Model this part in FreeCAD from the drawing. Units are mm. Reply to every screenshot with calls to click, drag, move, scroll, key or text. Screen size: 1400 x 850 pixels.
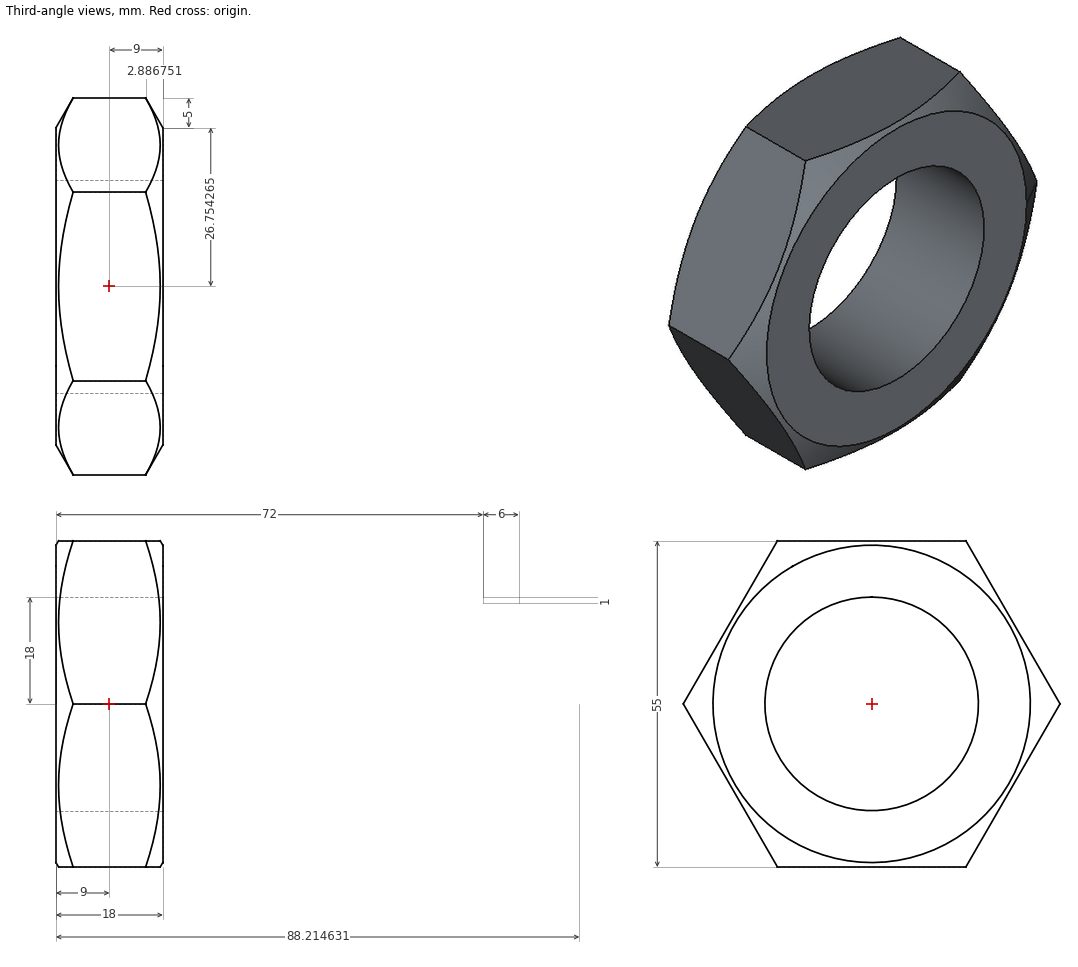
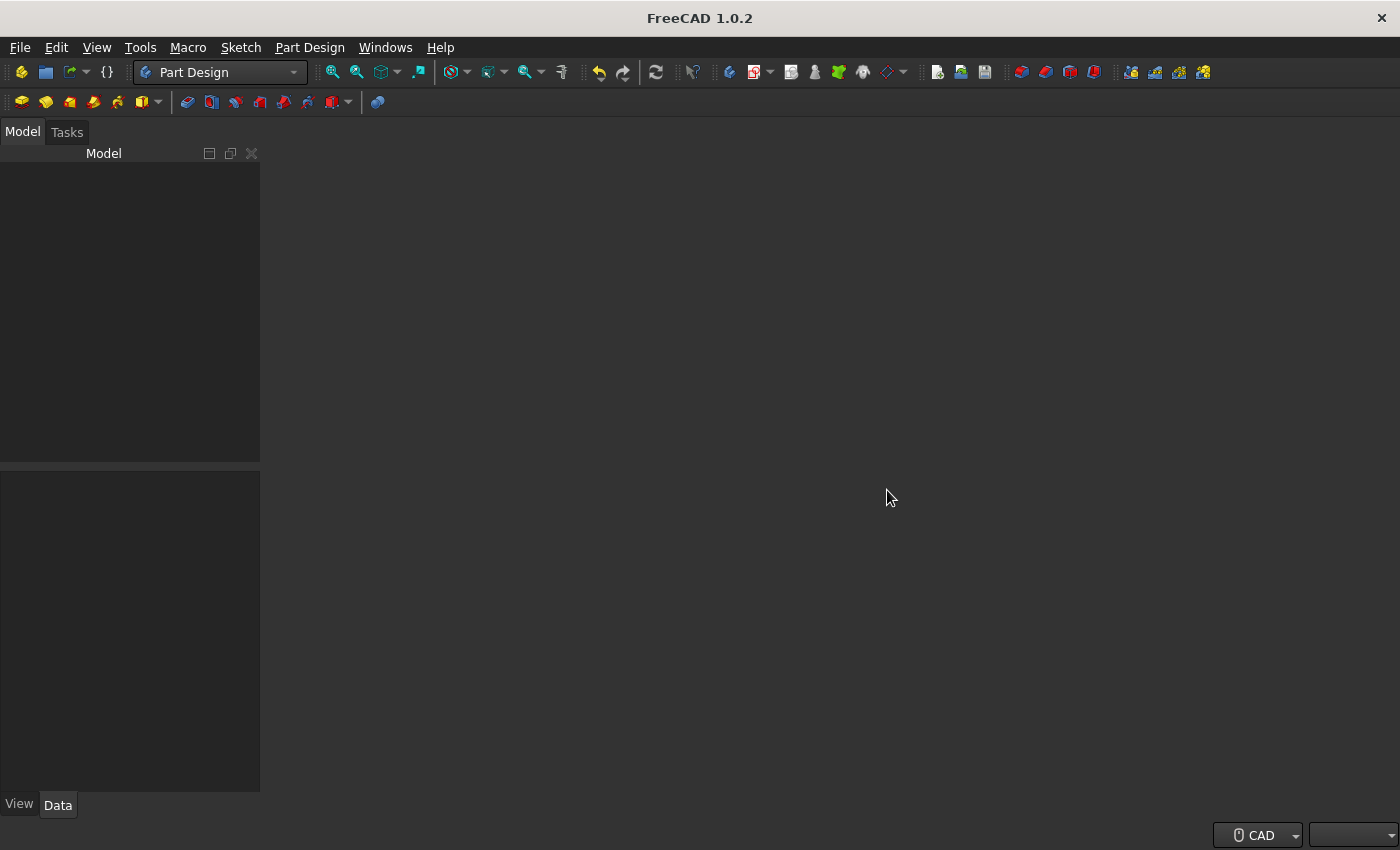
key(ctrl+n)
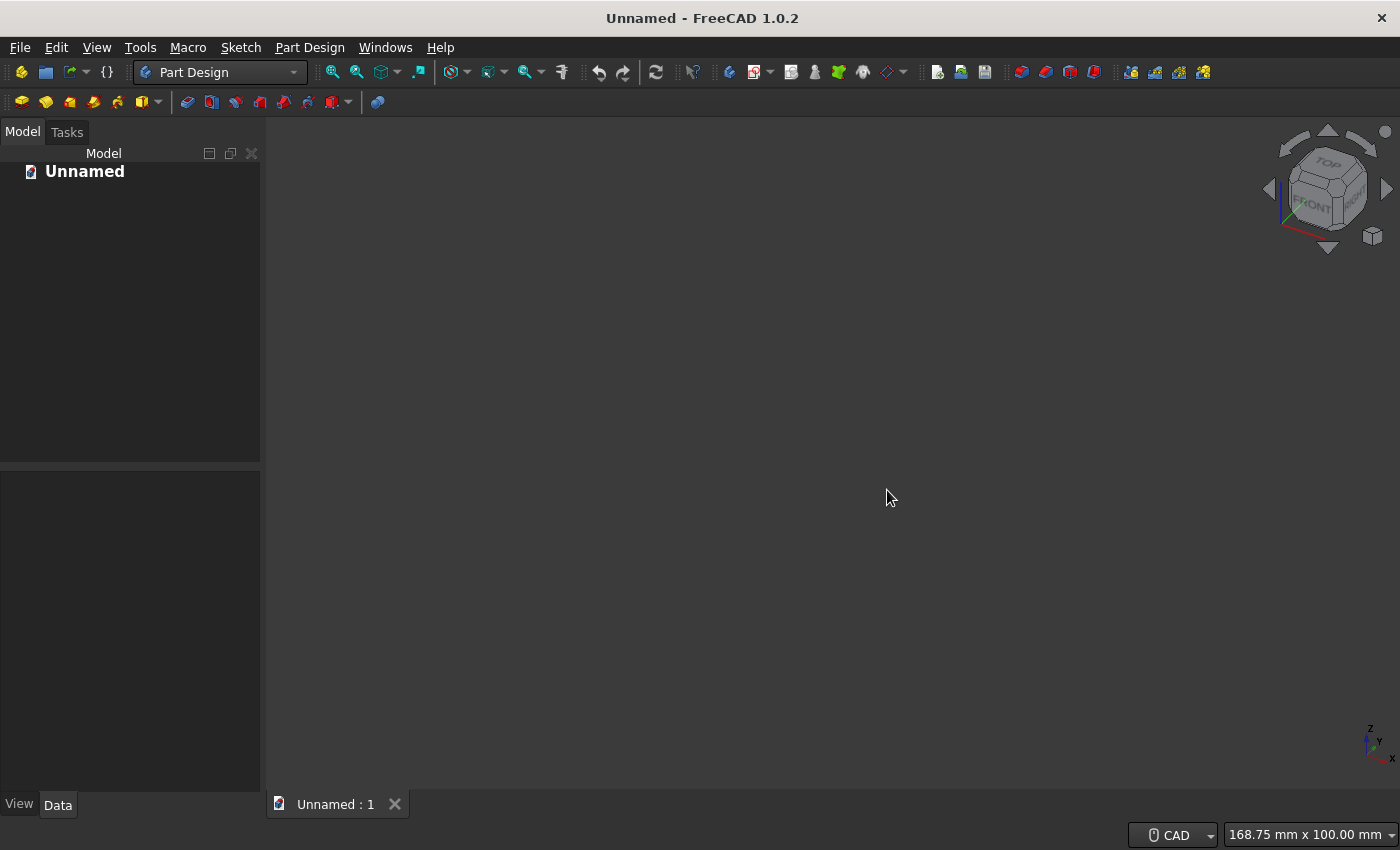
click(754, 72)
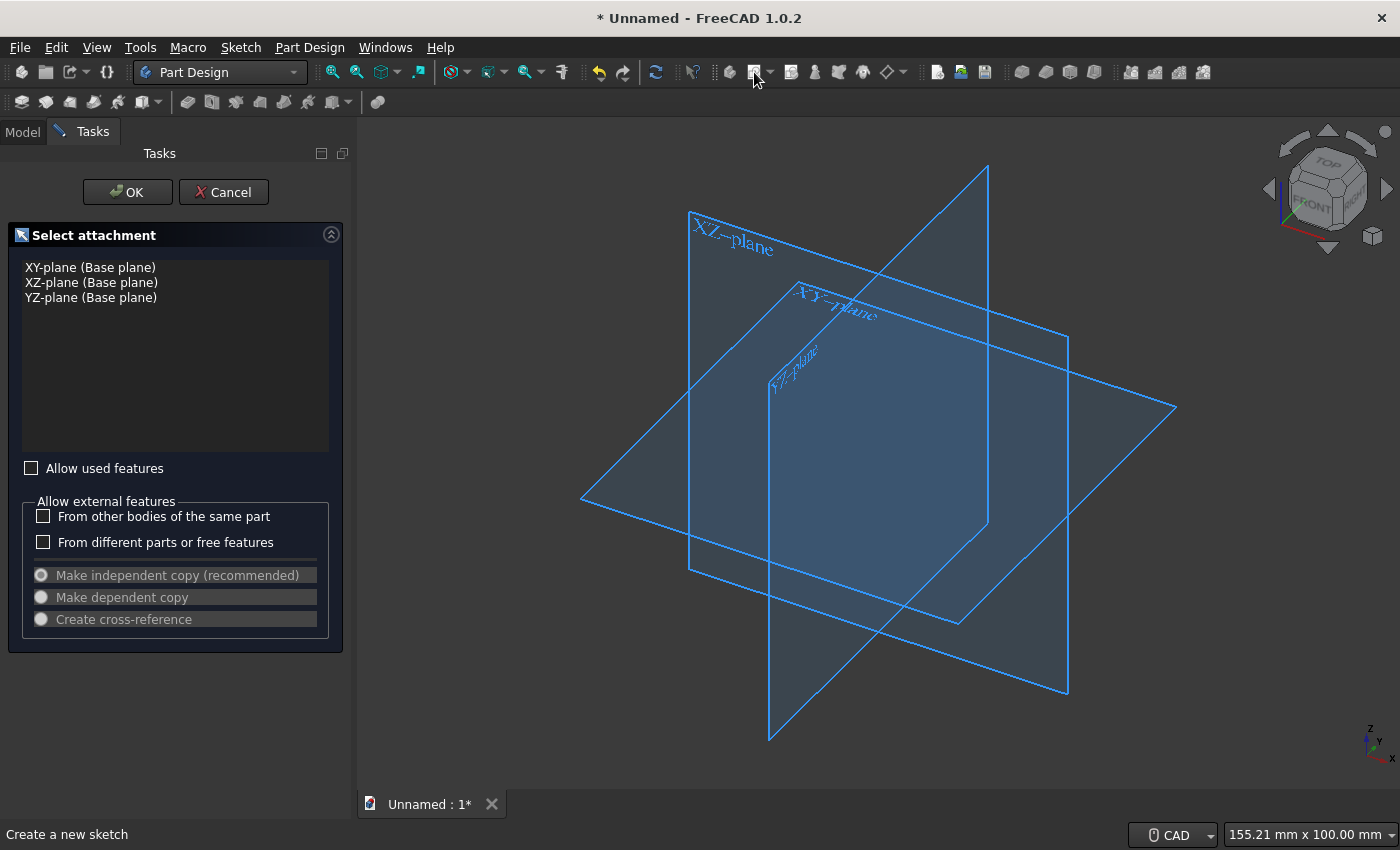
click(82, 298)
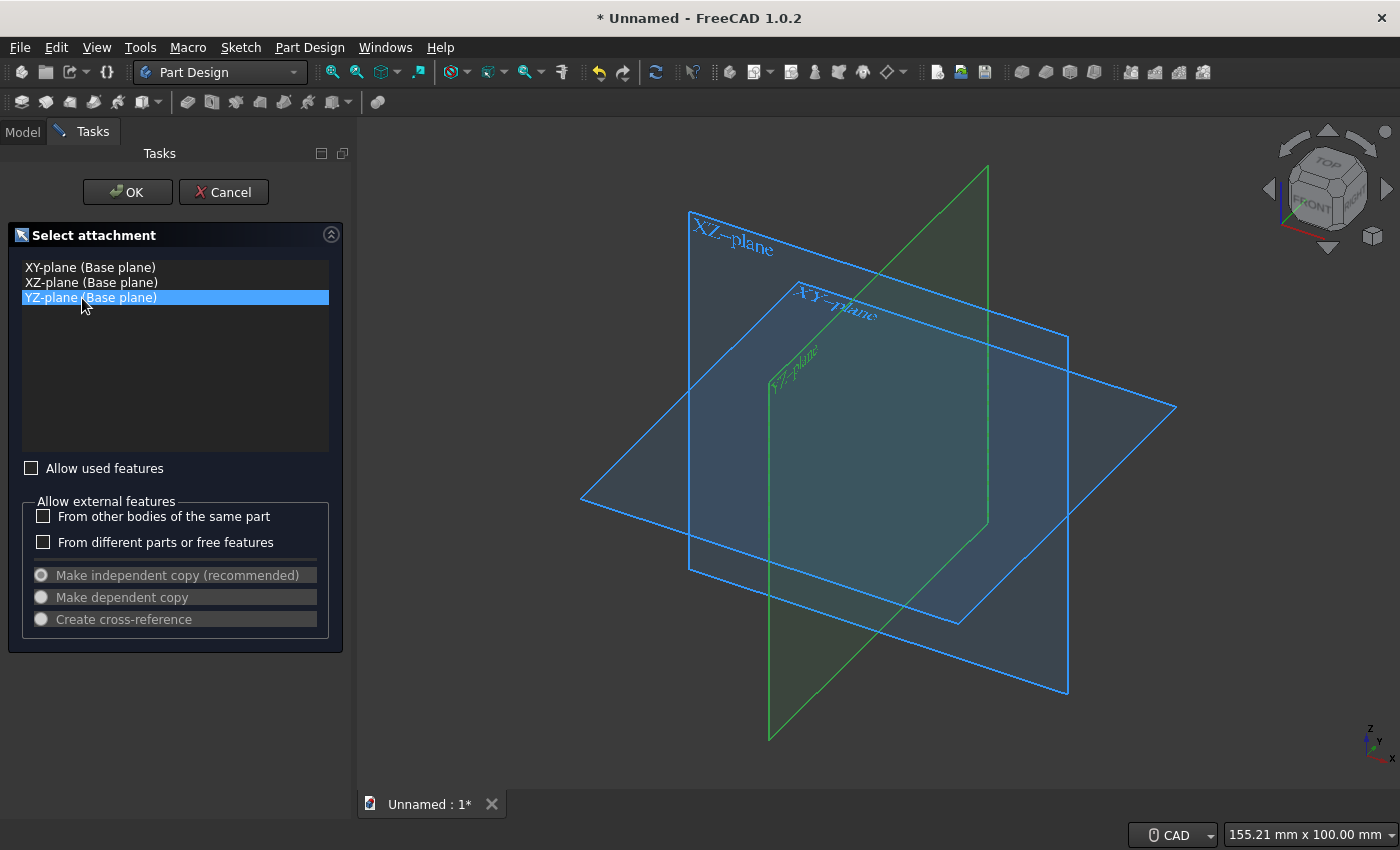
click(128, 192)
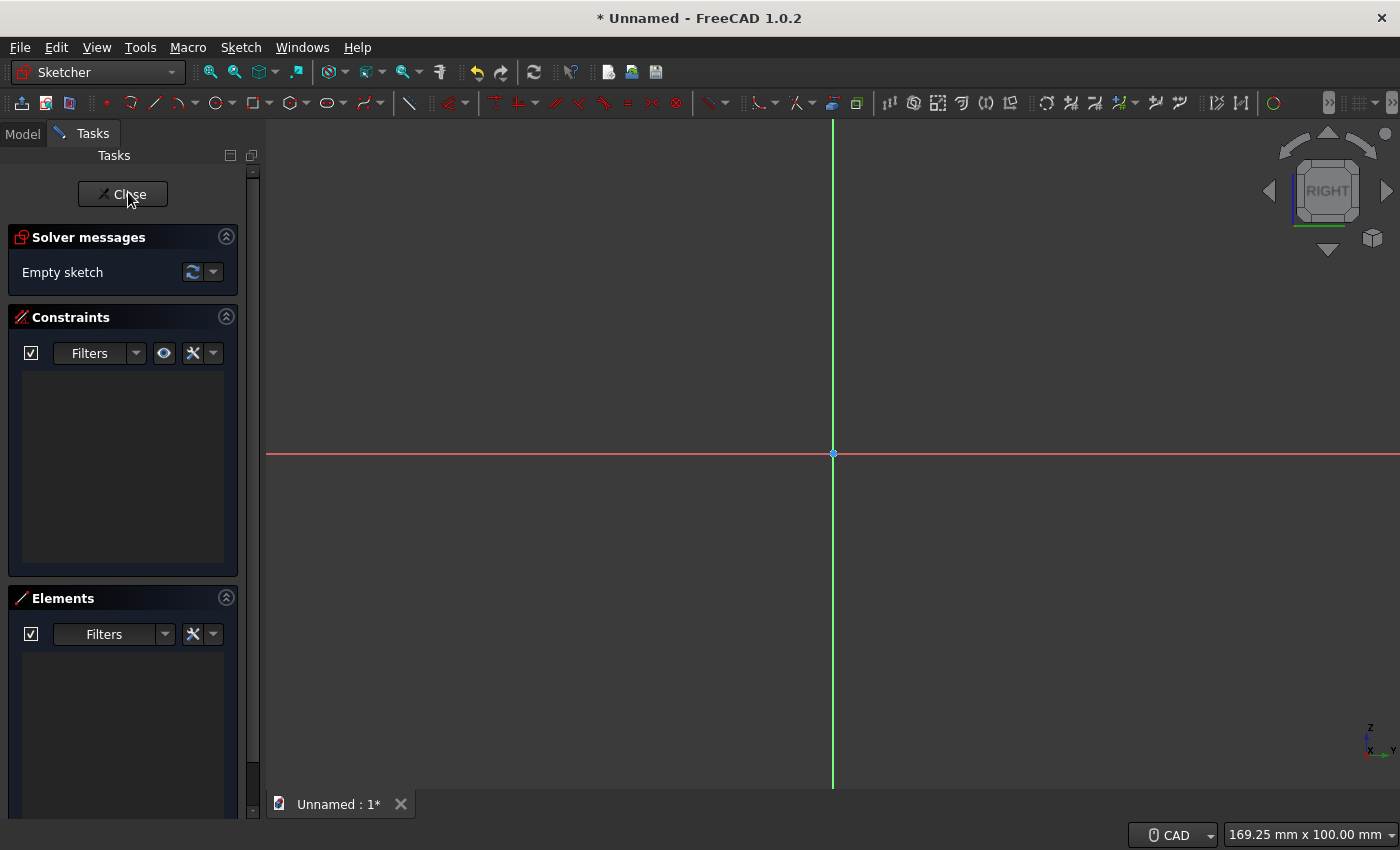
key(g)
key(p)
key(6)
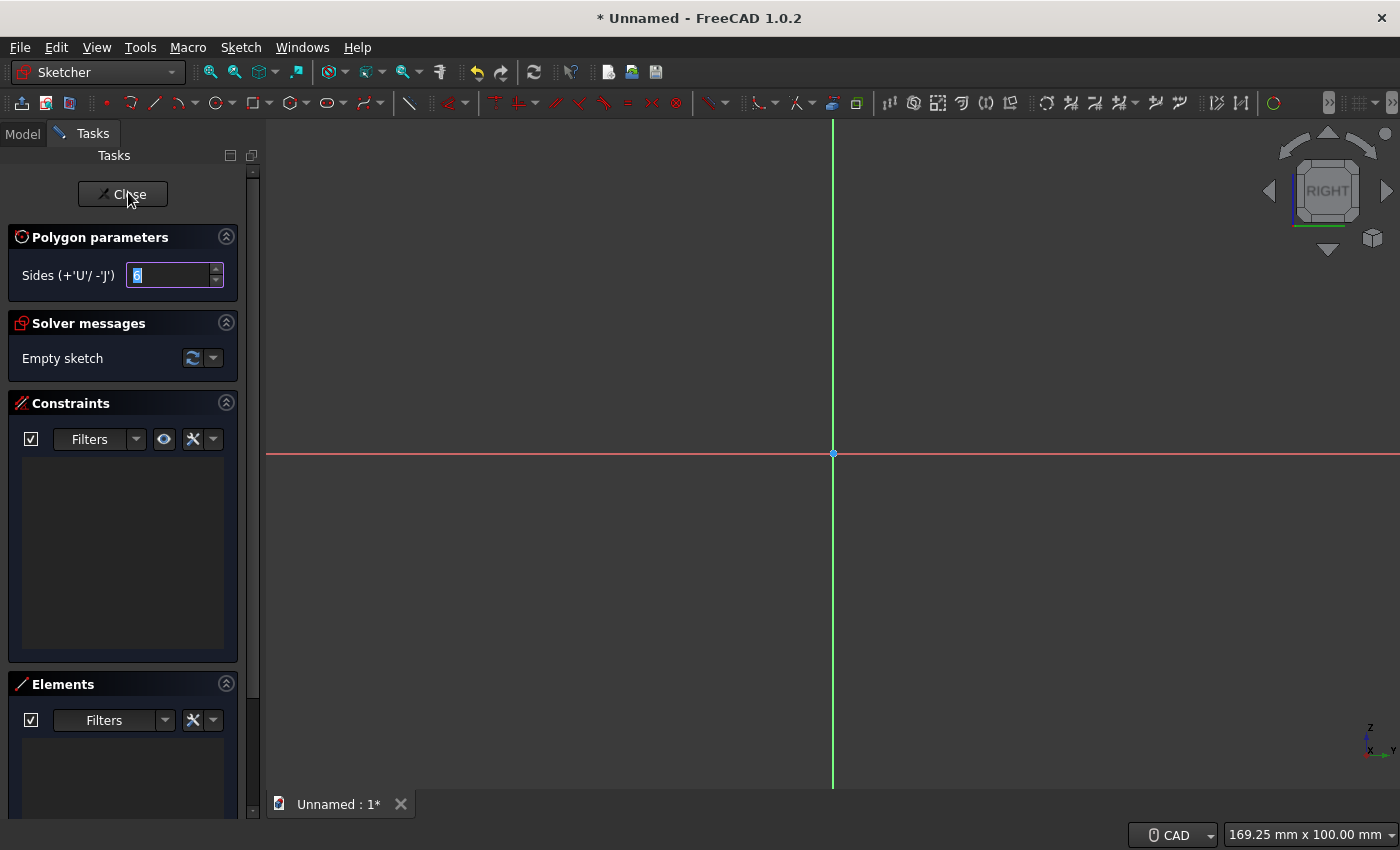
click(833, 454)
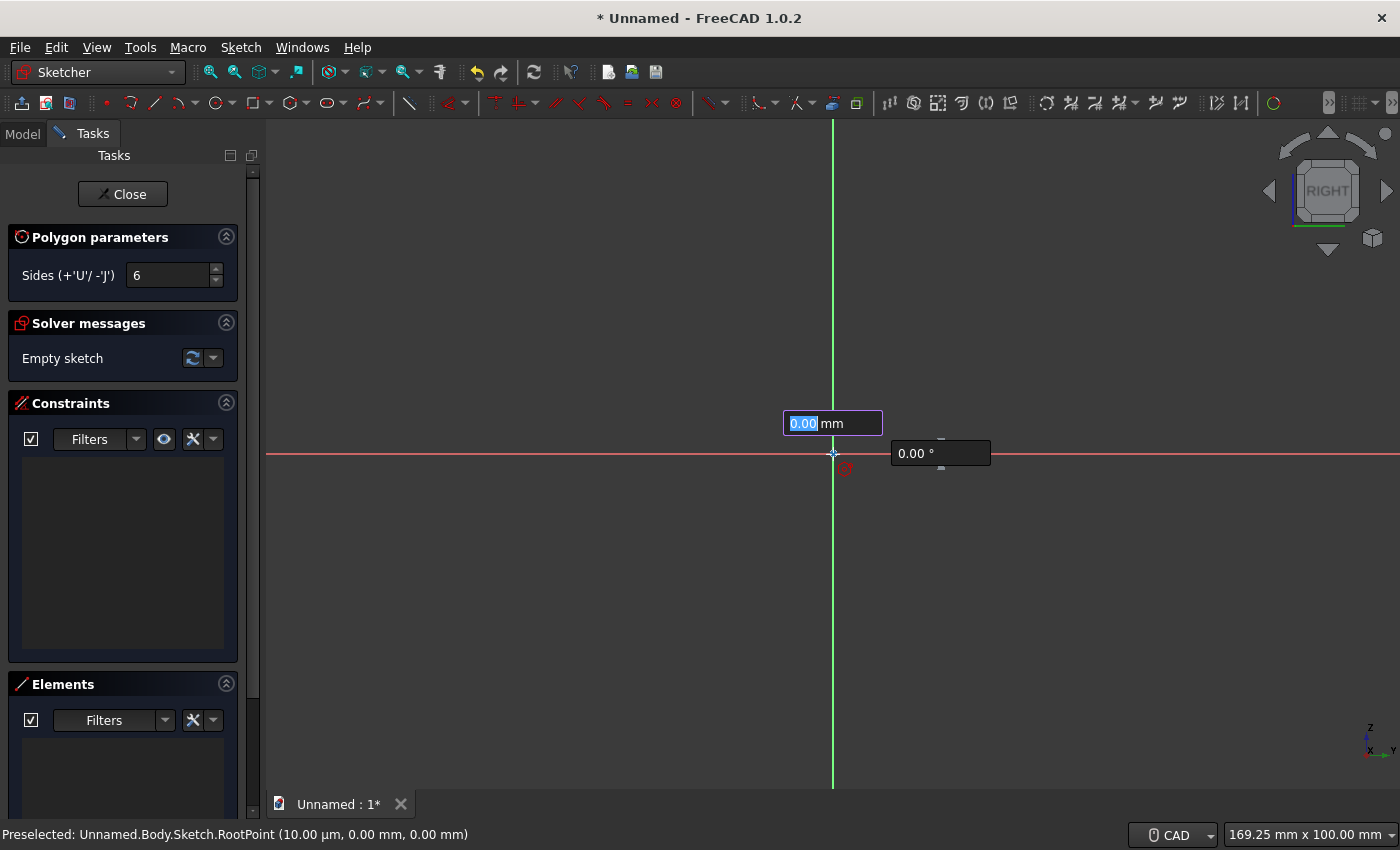
click(620, 454)
right_click(620, 454)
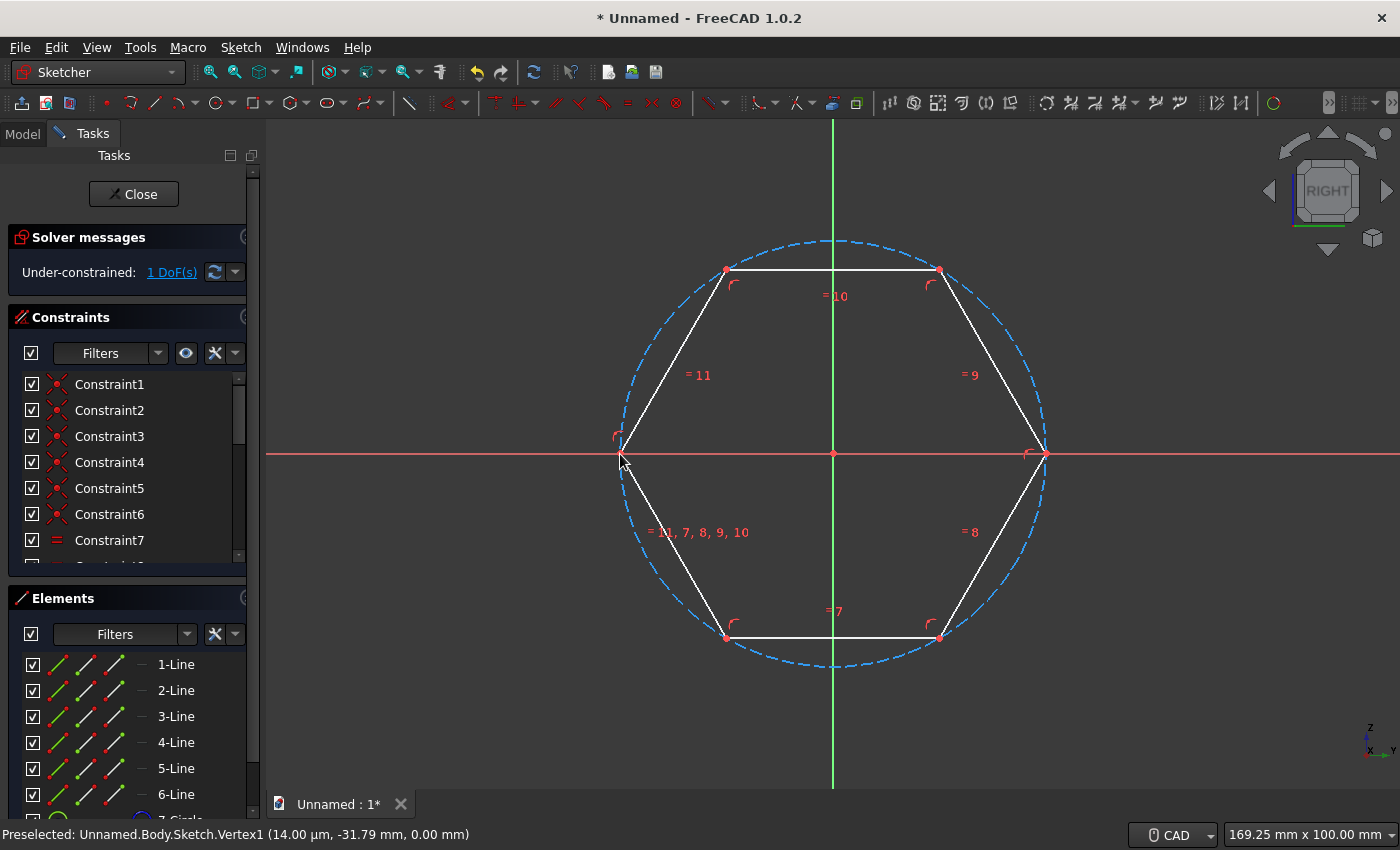
click(727, 638)